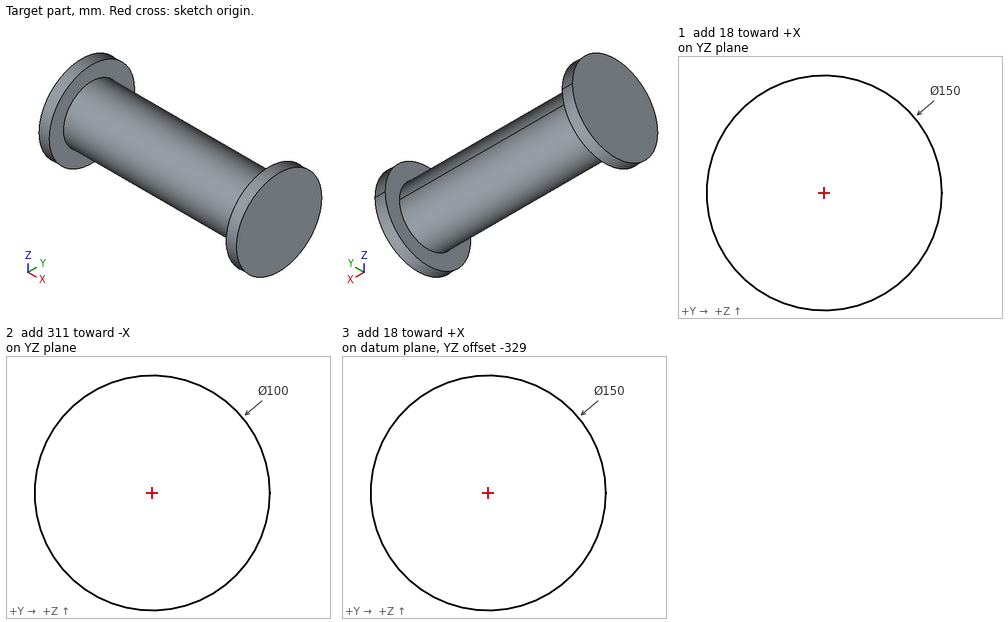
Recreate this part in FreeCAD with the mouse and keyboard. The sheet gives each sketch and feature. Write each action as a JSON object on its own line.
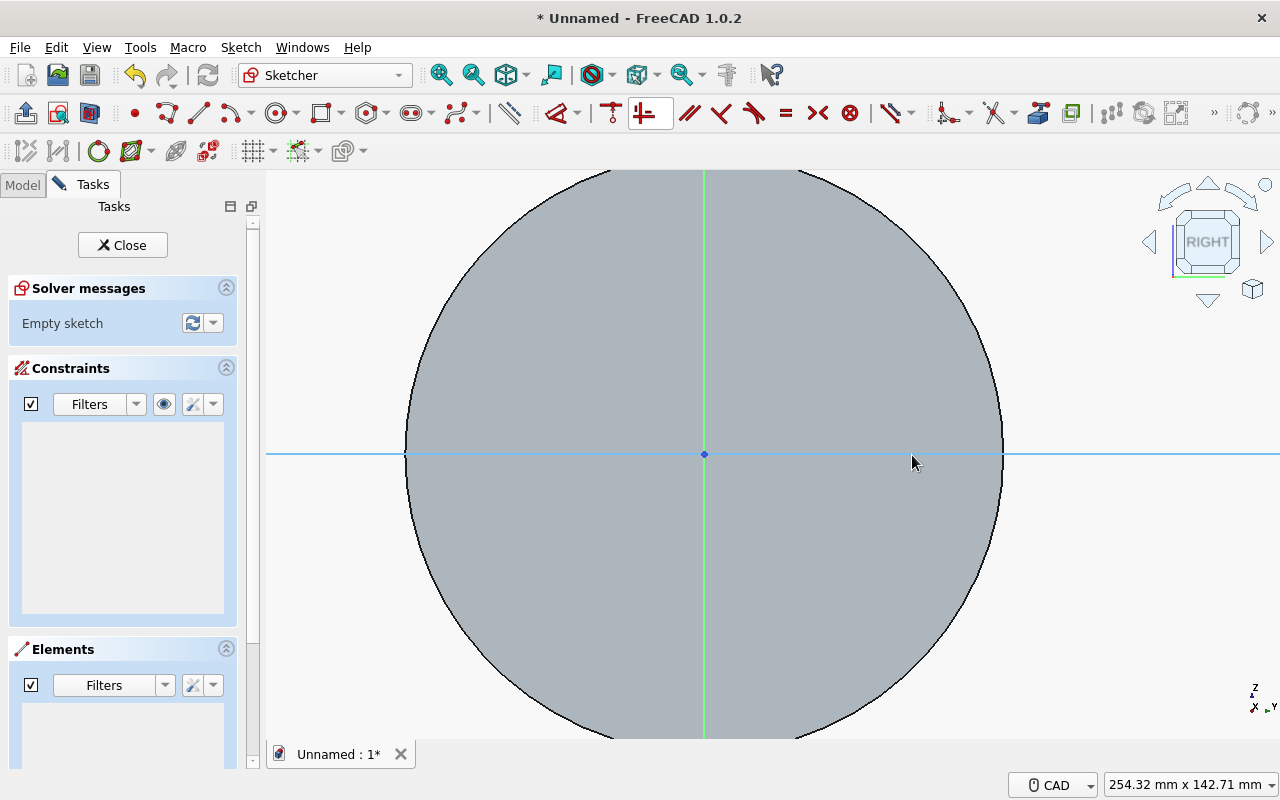
{"action": "left_click", "coordinate": [276, 114]}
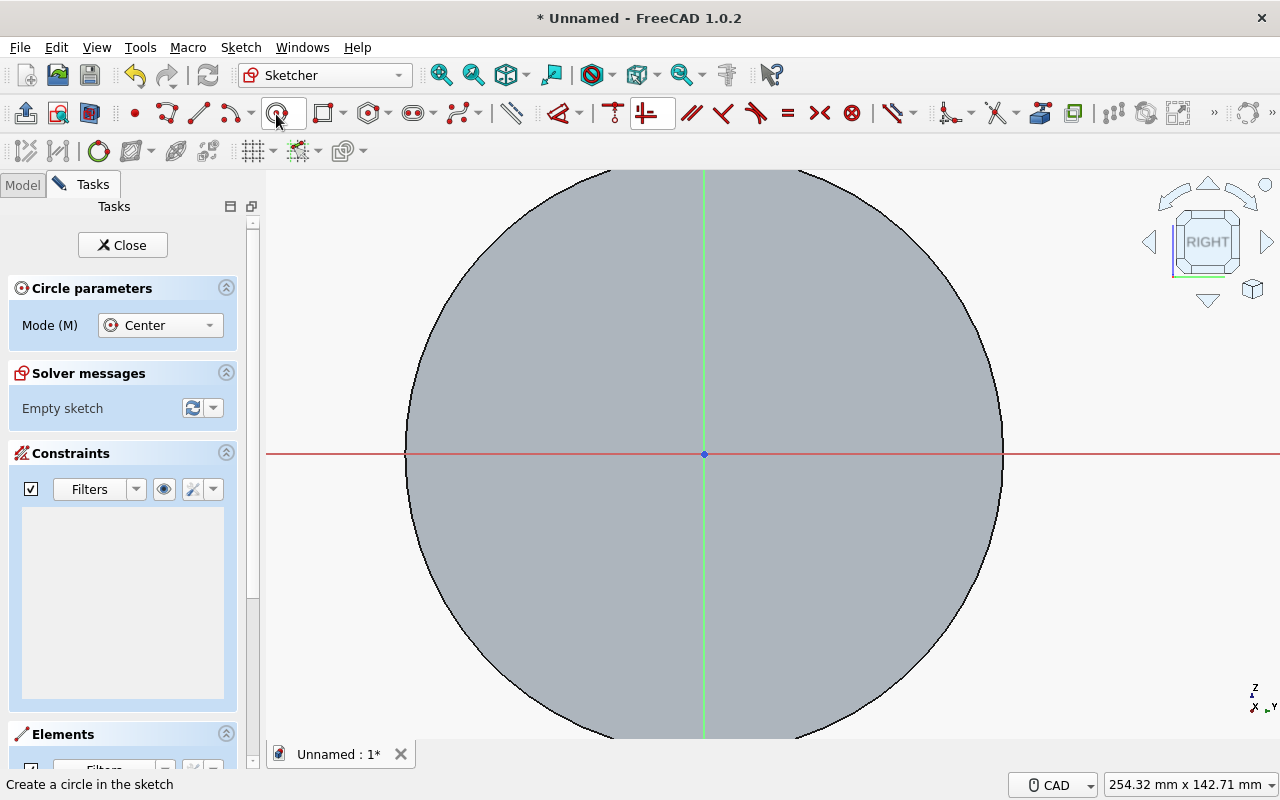
{"action": "left_click", "coordinate": [704, 454]}
{"action": "left_click", "coordinate": [845, 313]}
{"action": "key", "text": "Escape"}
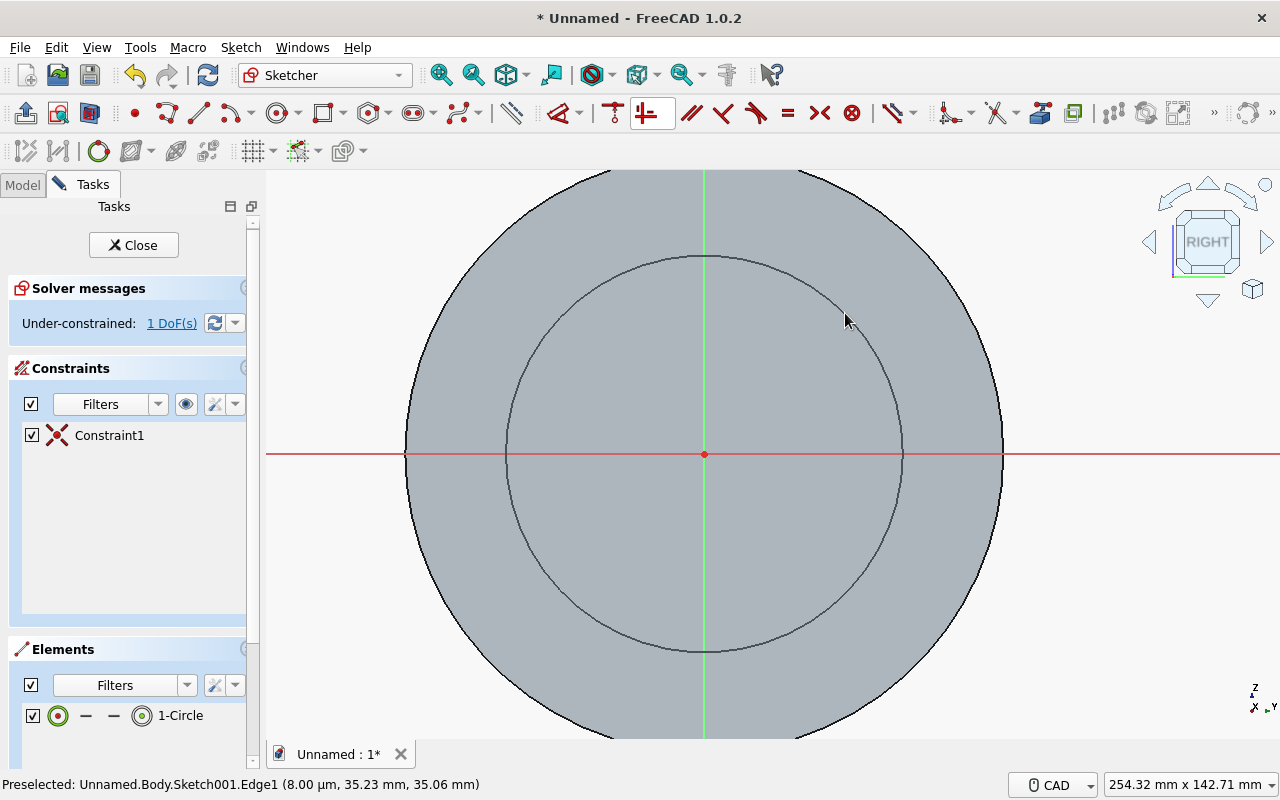
{"action": "left_click", "coordinate": [844, 313]}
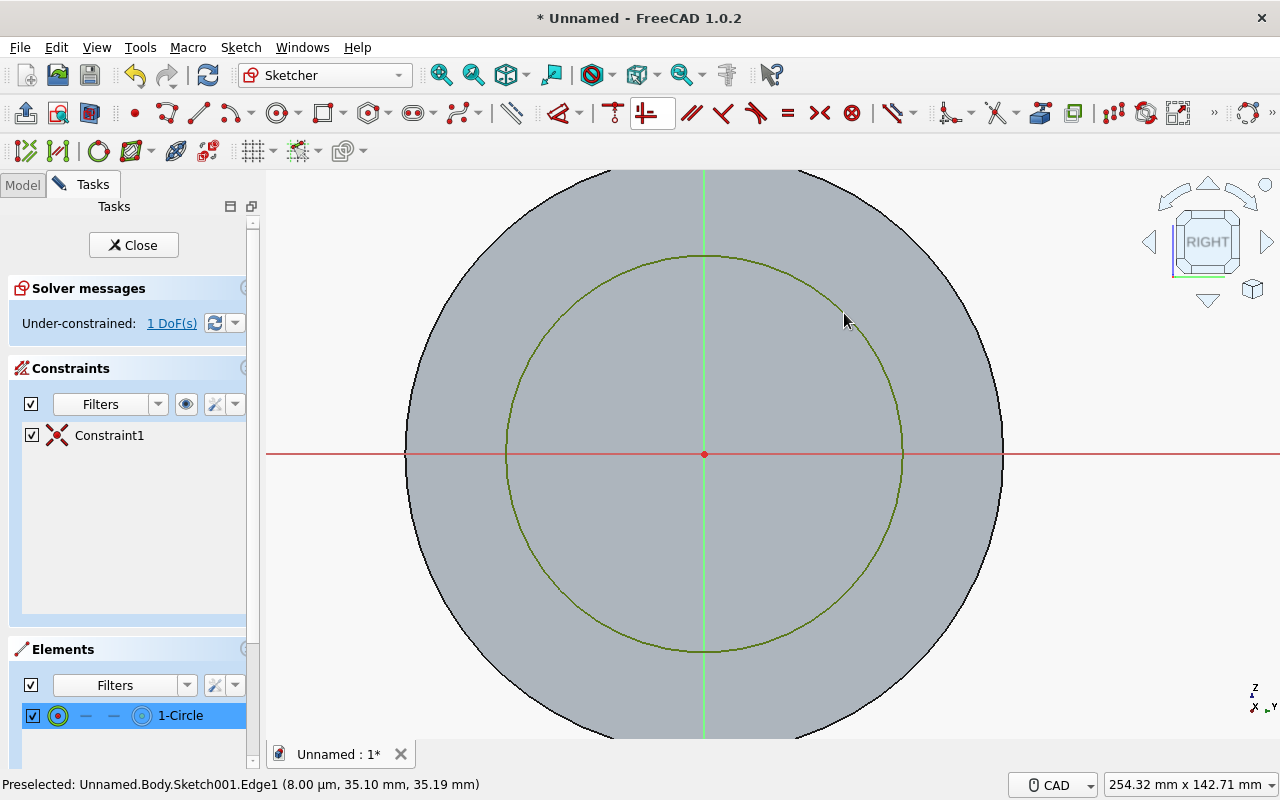
{"action": "left_click", "coordinate": [582, 114]}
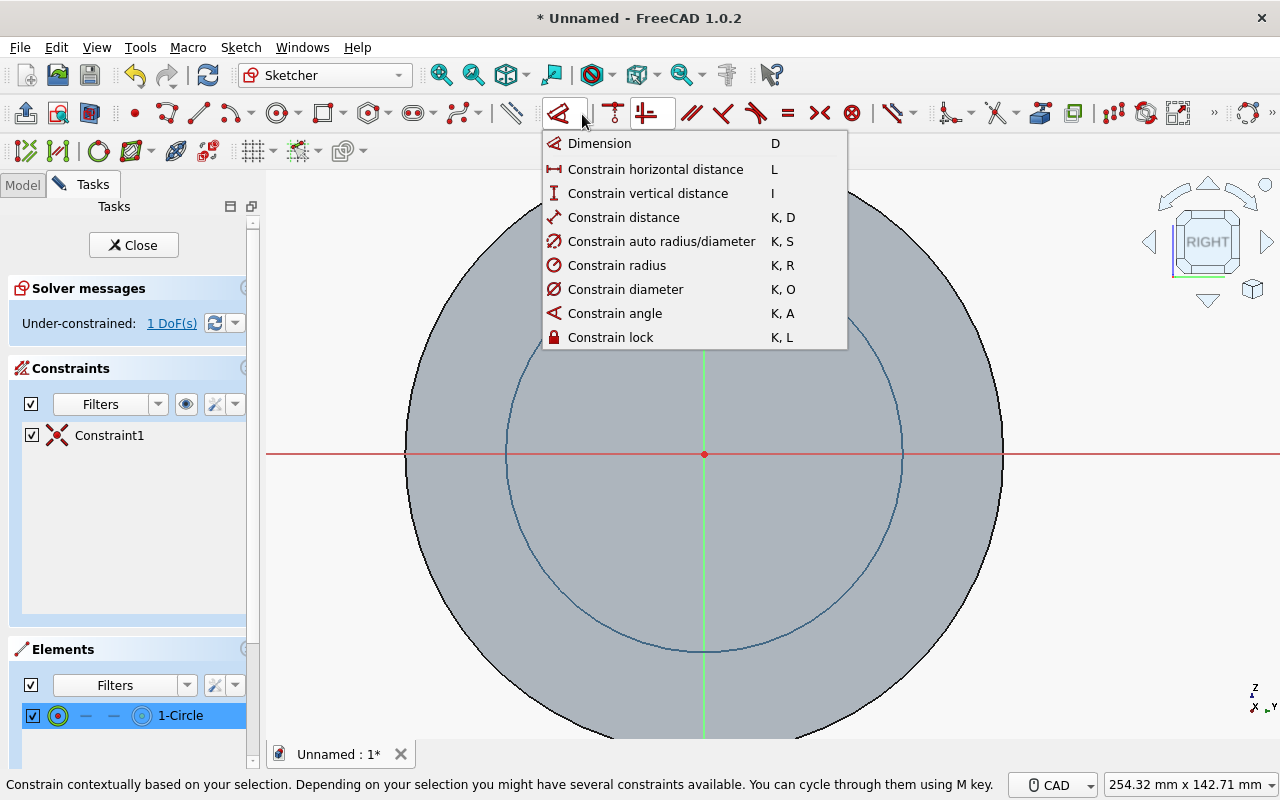
{"action": "left_click", "coordinate": [695, 289]}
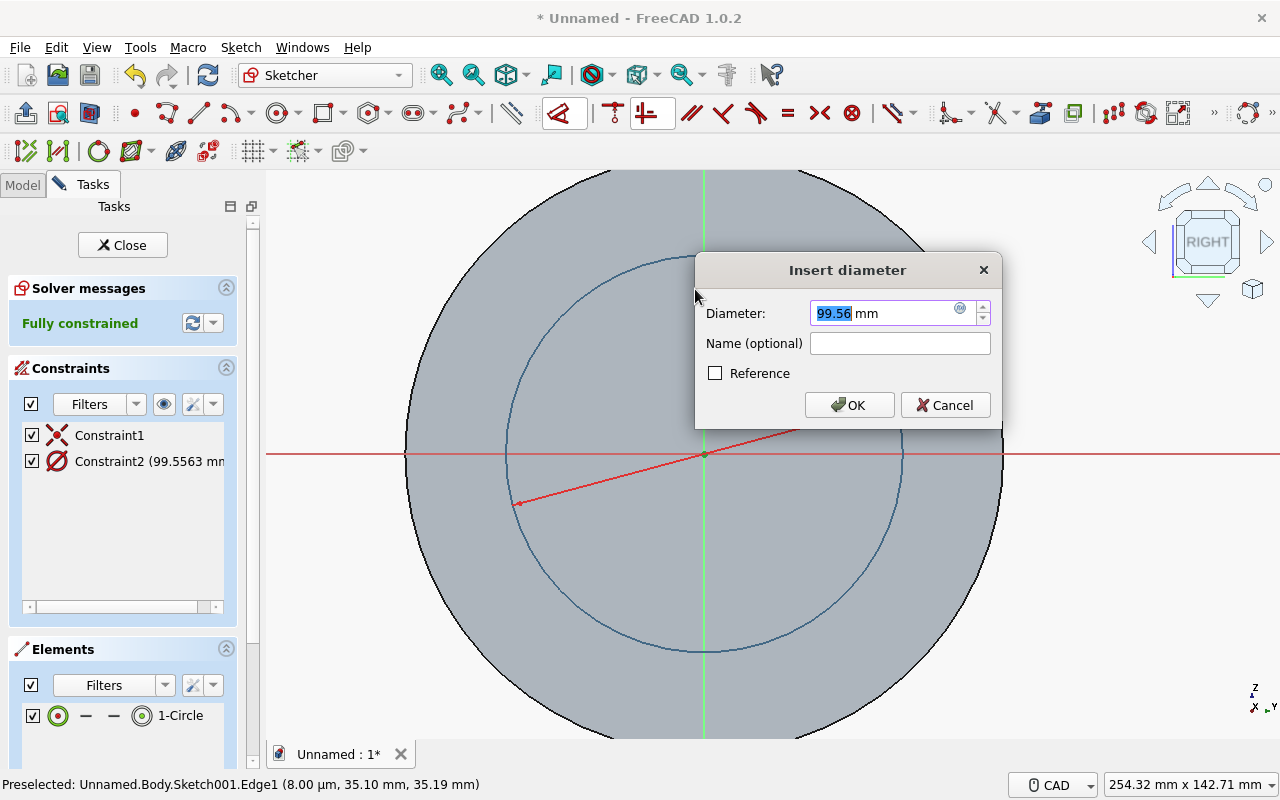
{"action": "type", "text": "100"}
{"action": "key", "text": "Return"}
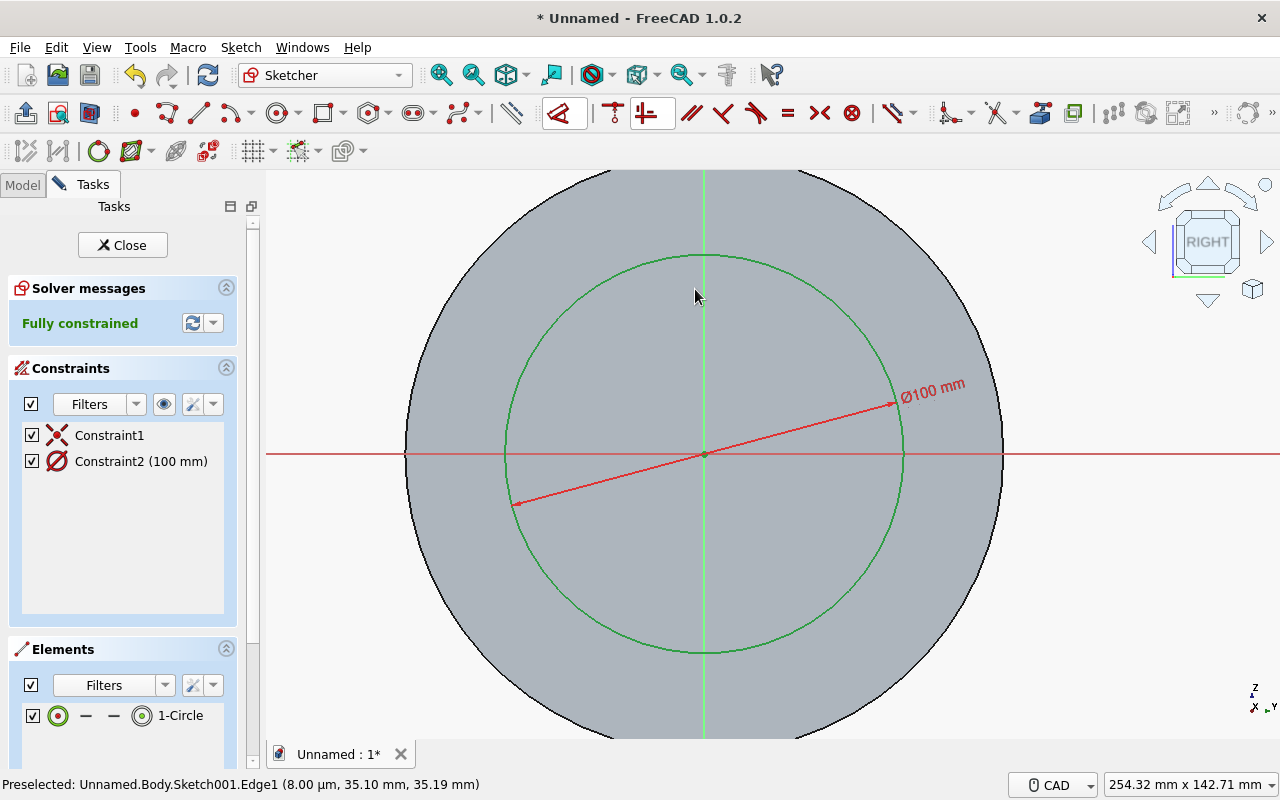
{"action": "left_click", "coordinate": [123, 245]}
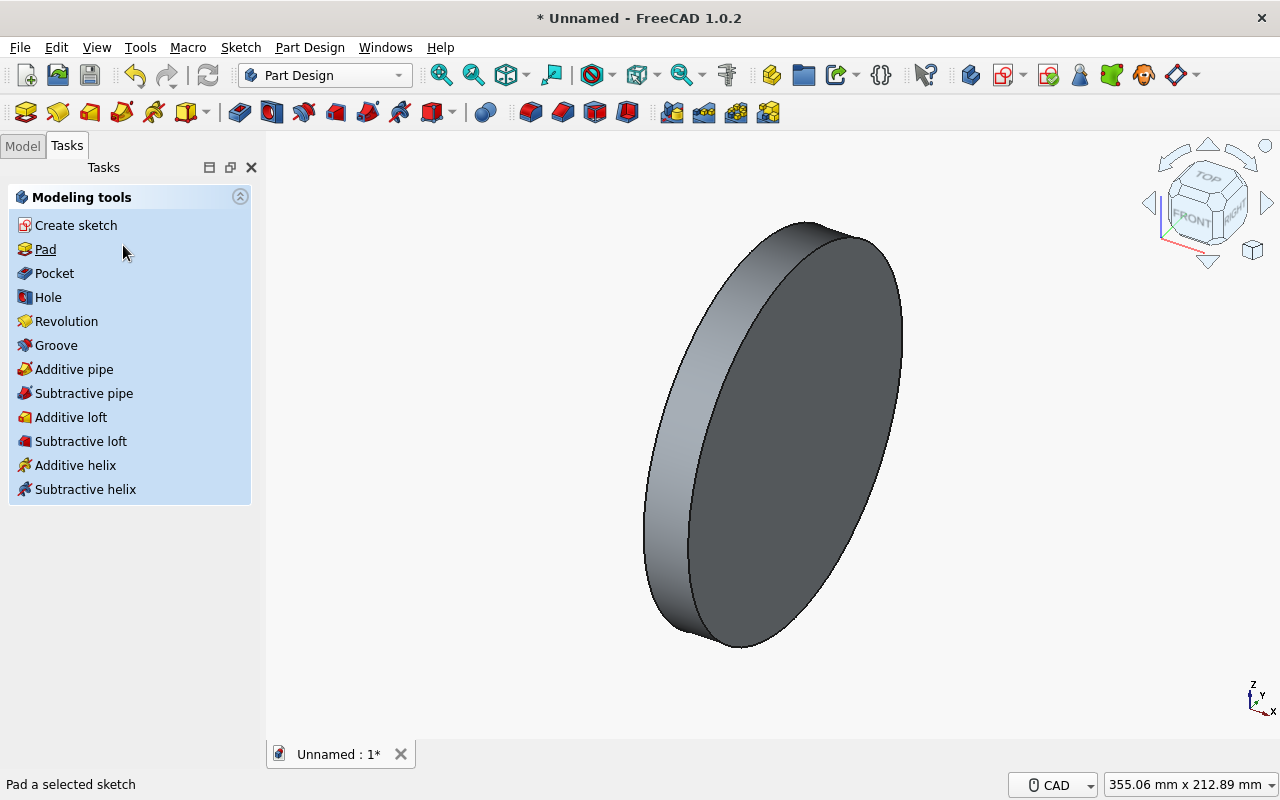
{"action": "left_click", "coordinate": [26, 112]}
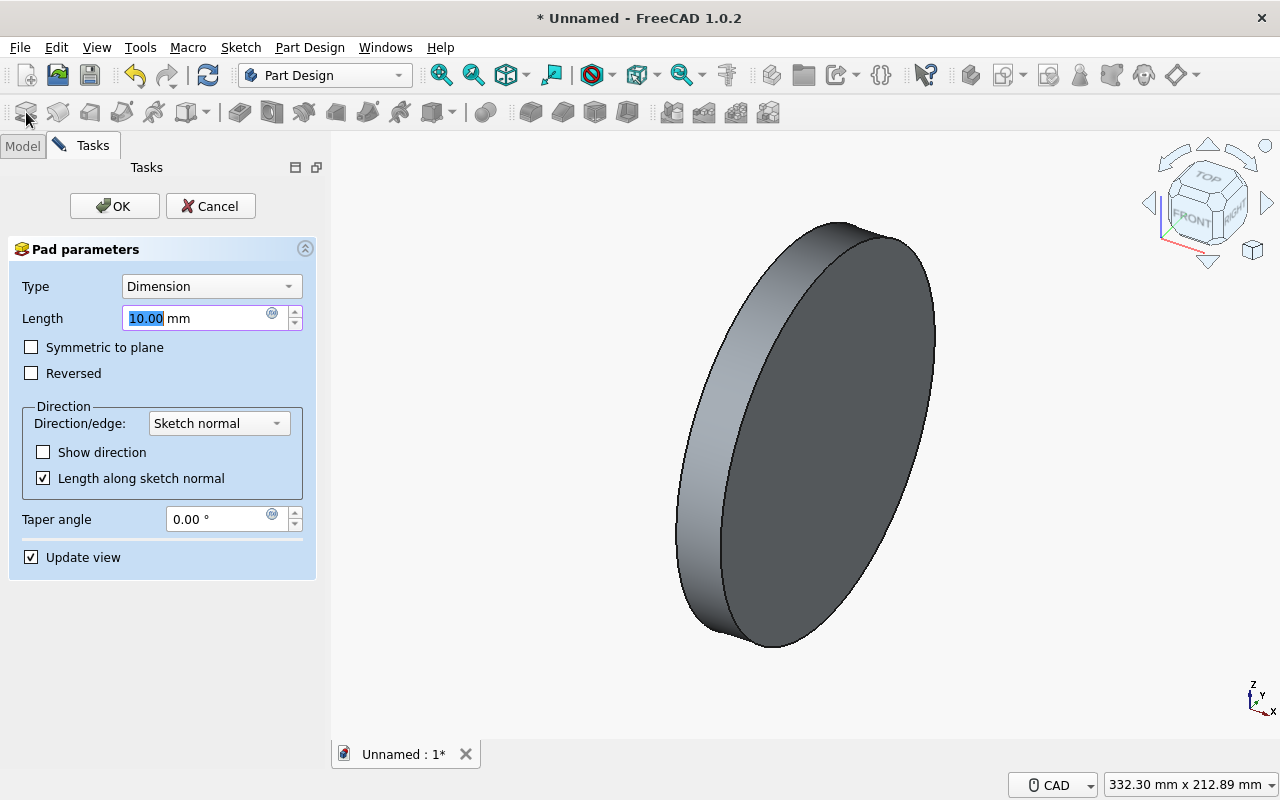
{"action": "type", "text": "311"}
{"action": "key", "text": "Tab"}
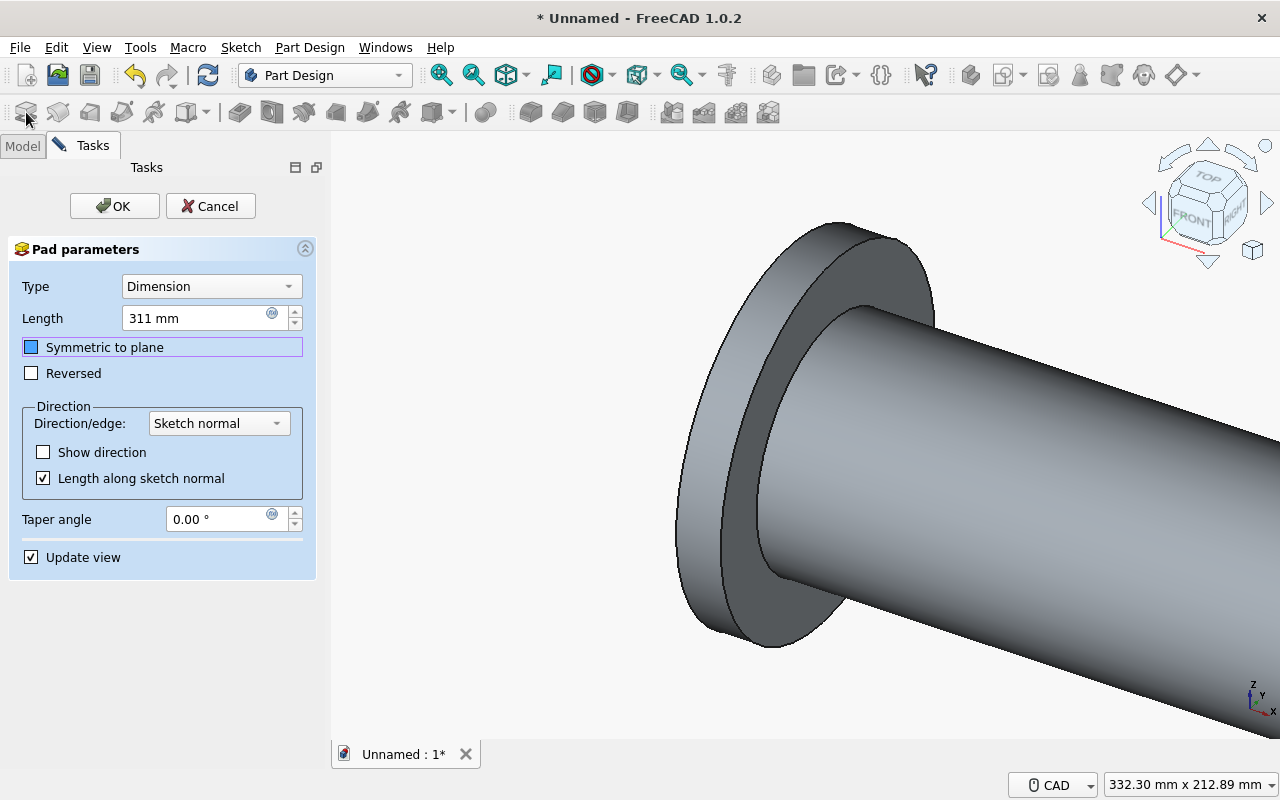
{"action": "left_click", "coordinate": [30, 373]}